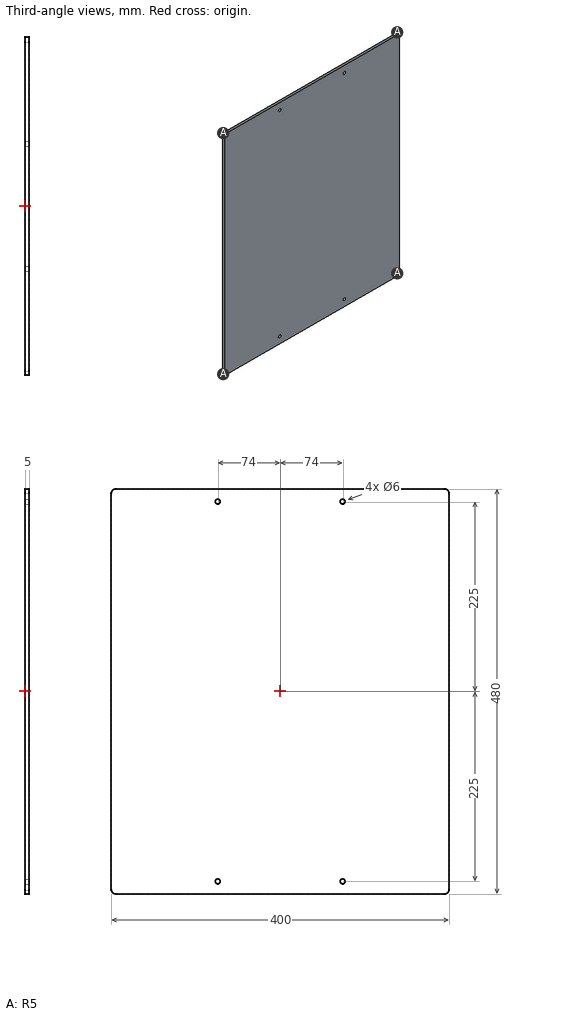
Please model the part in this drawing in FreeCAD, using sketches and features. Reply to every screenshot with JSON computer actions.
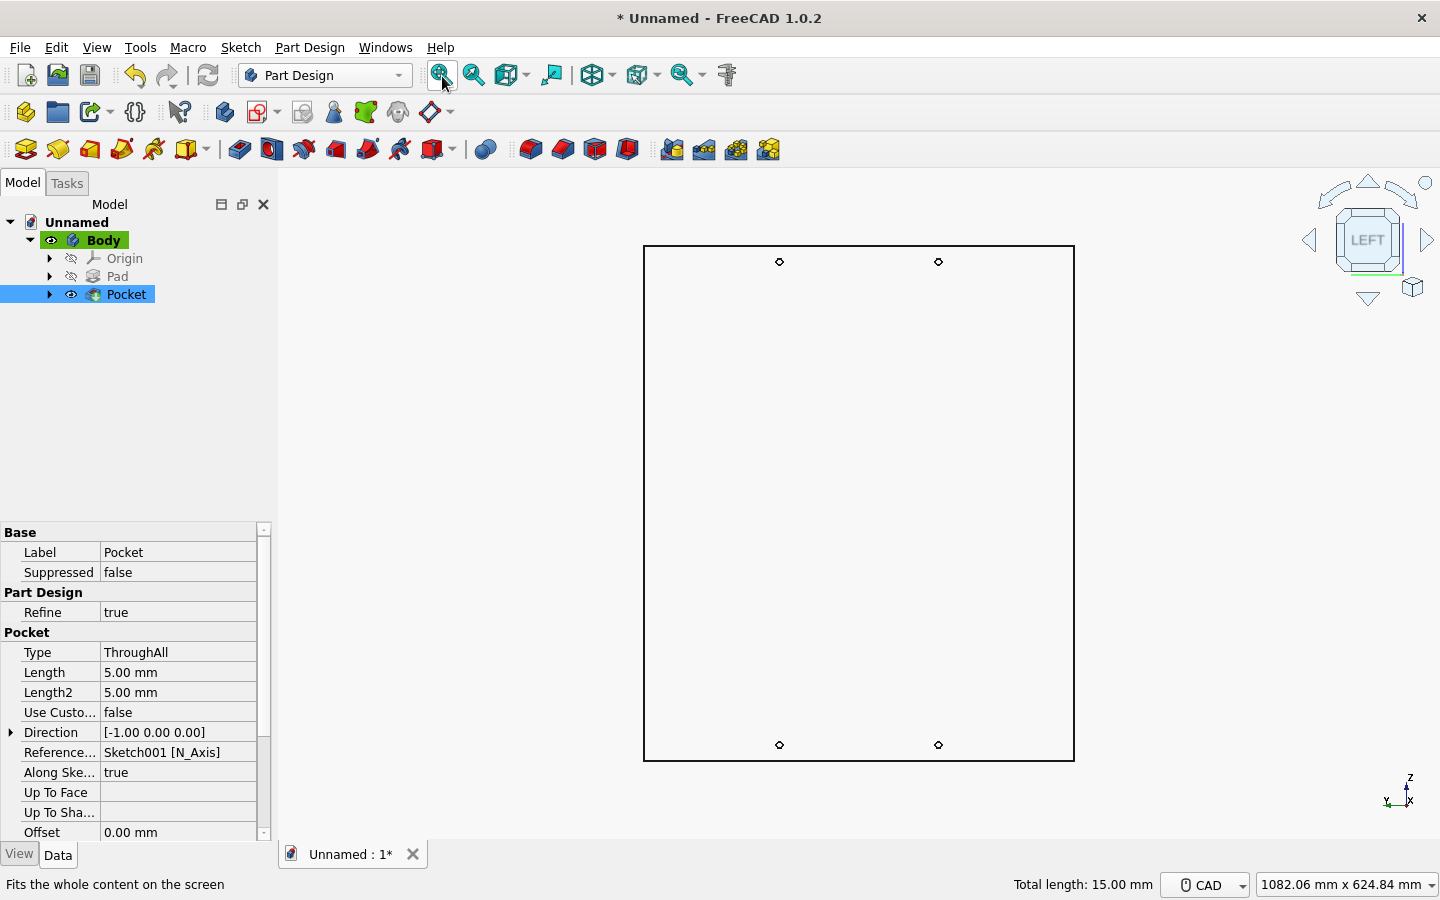
{"action": "key", "text": "0"}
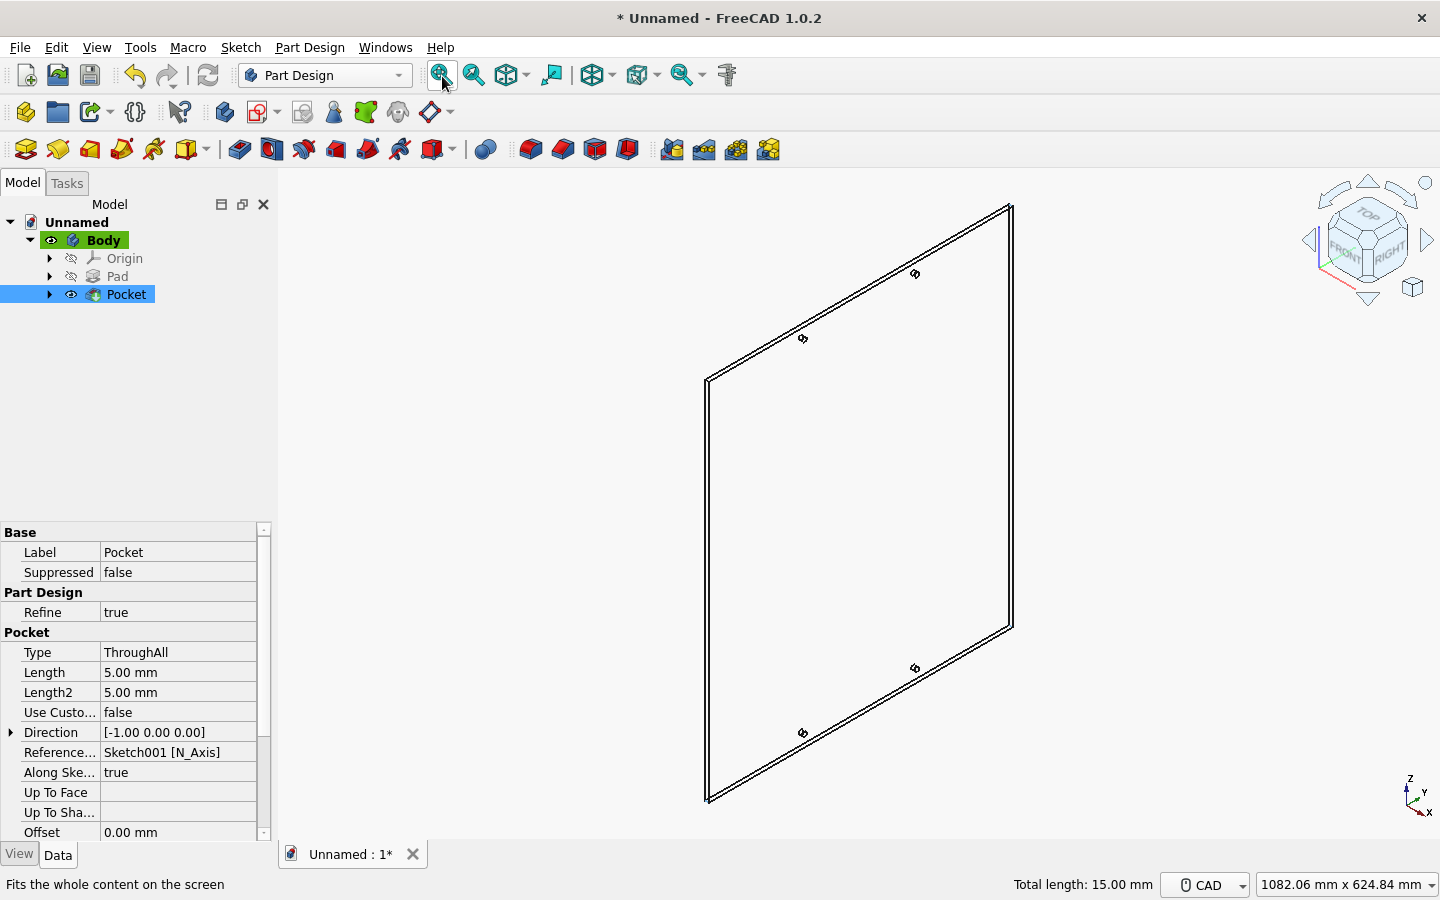
{"action": "scroll", "coordinate": [707, 380], "scroll_direction": "up", "scroll_amount": 11}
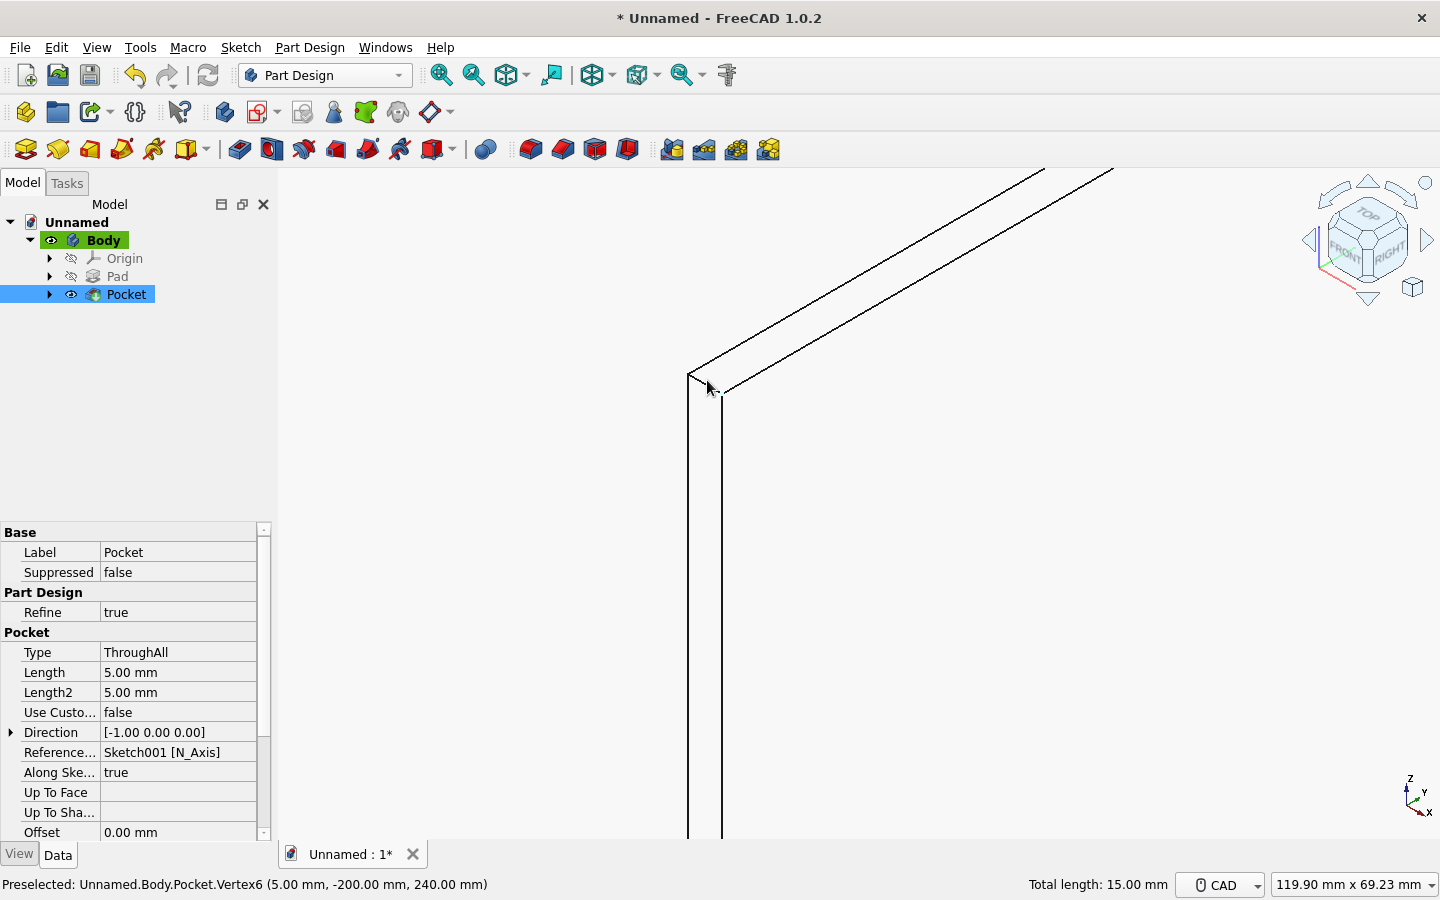
{"action": "left_click", "coordinate": [705, 383], "text": "ctrl"}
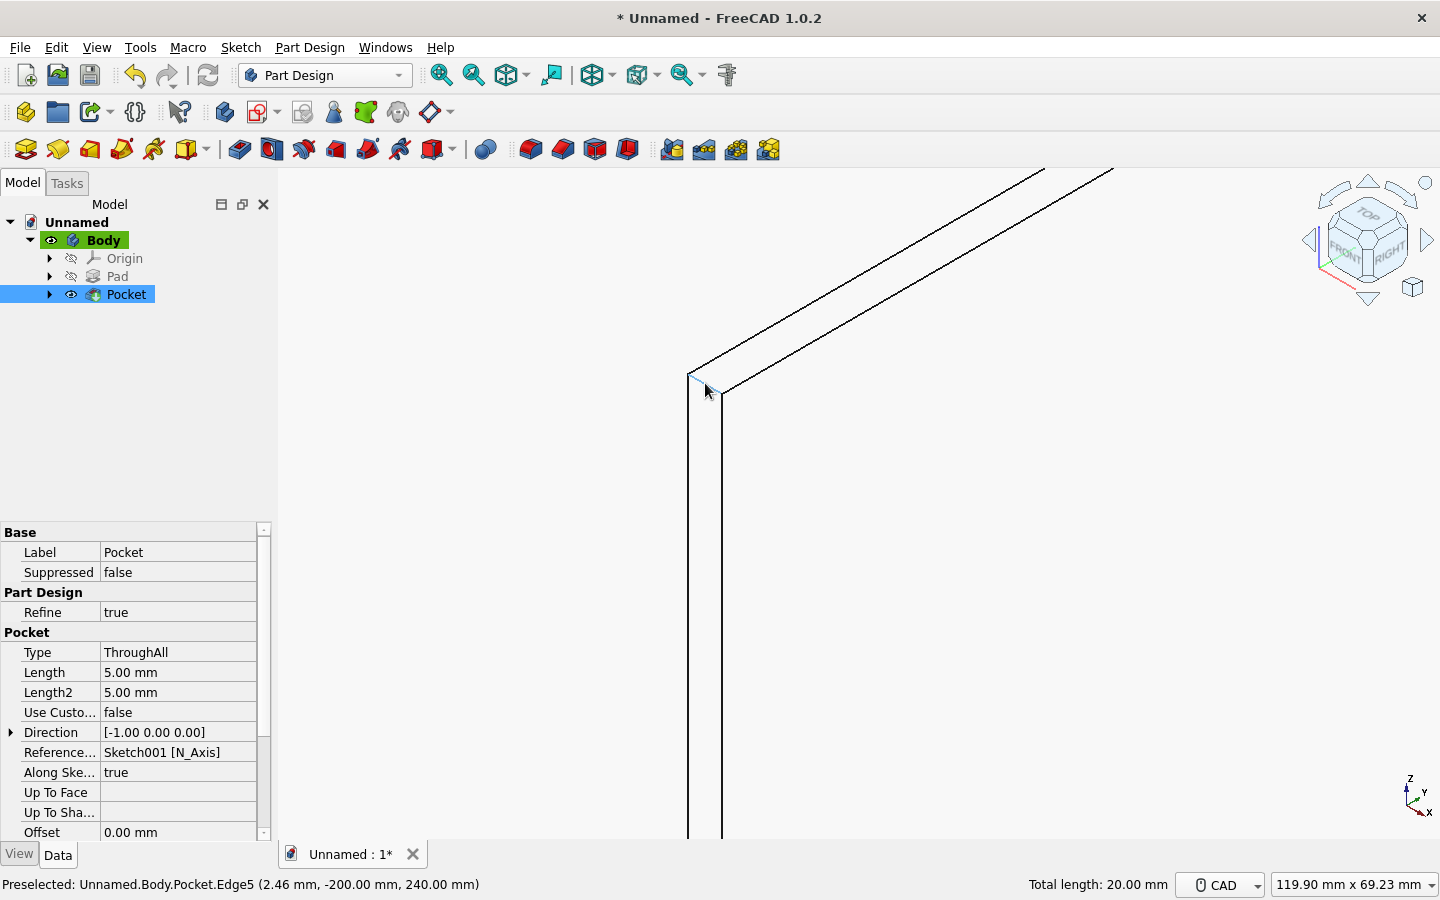
{"action": "key", "text": "v 1"}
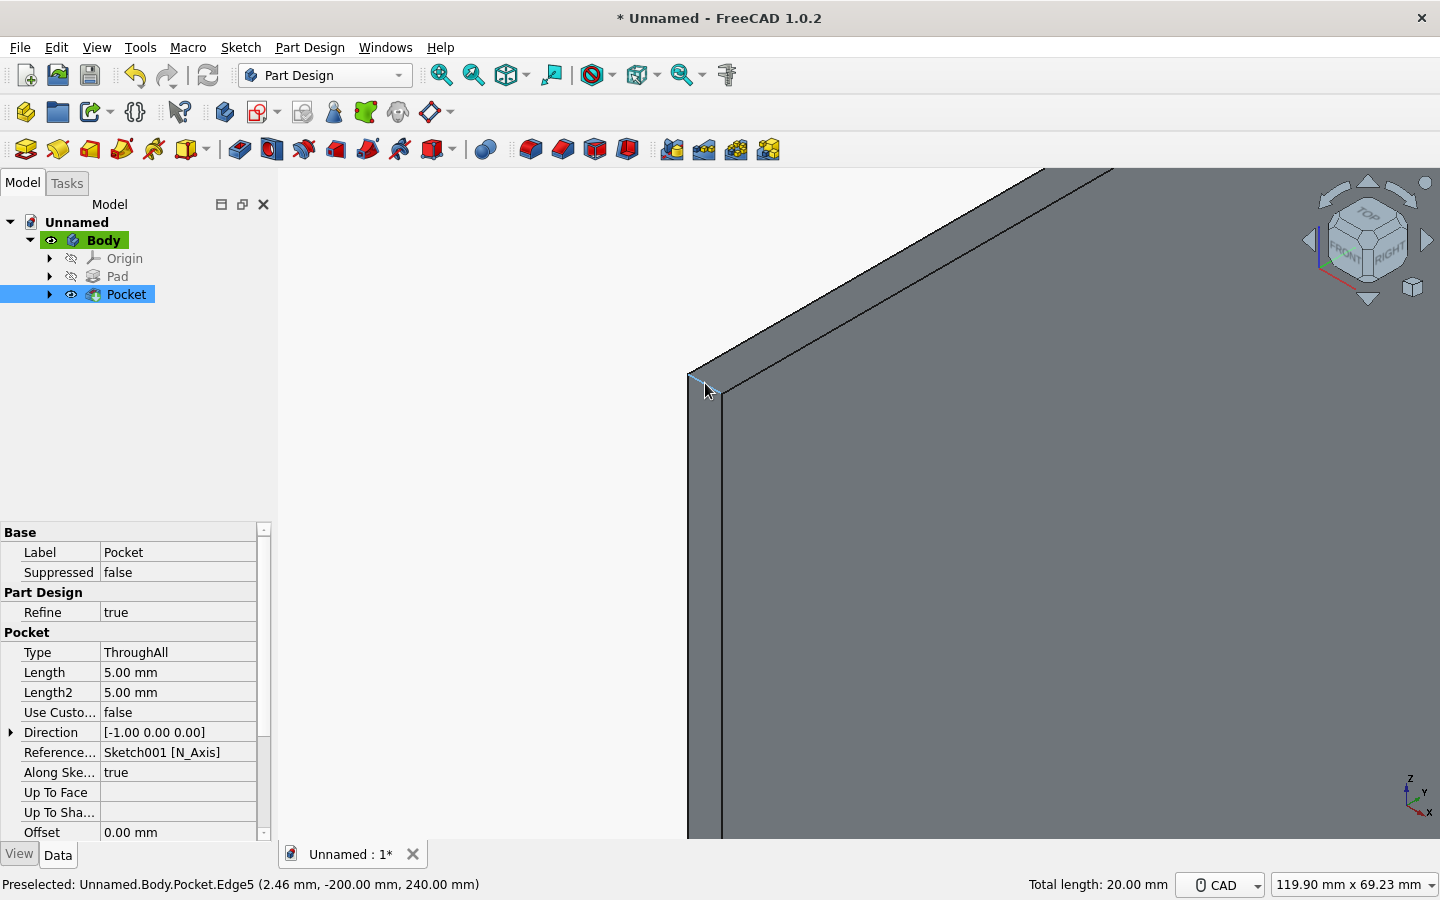
{"action": "left_click", "coordinate": [532, 150]}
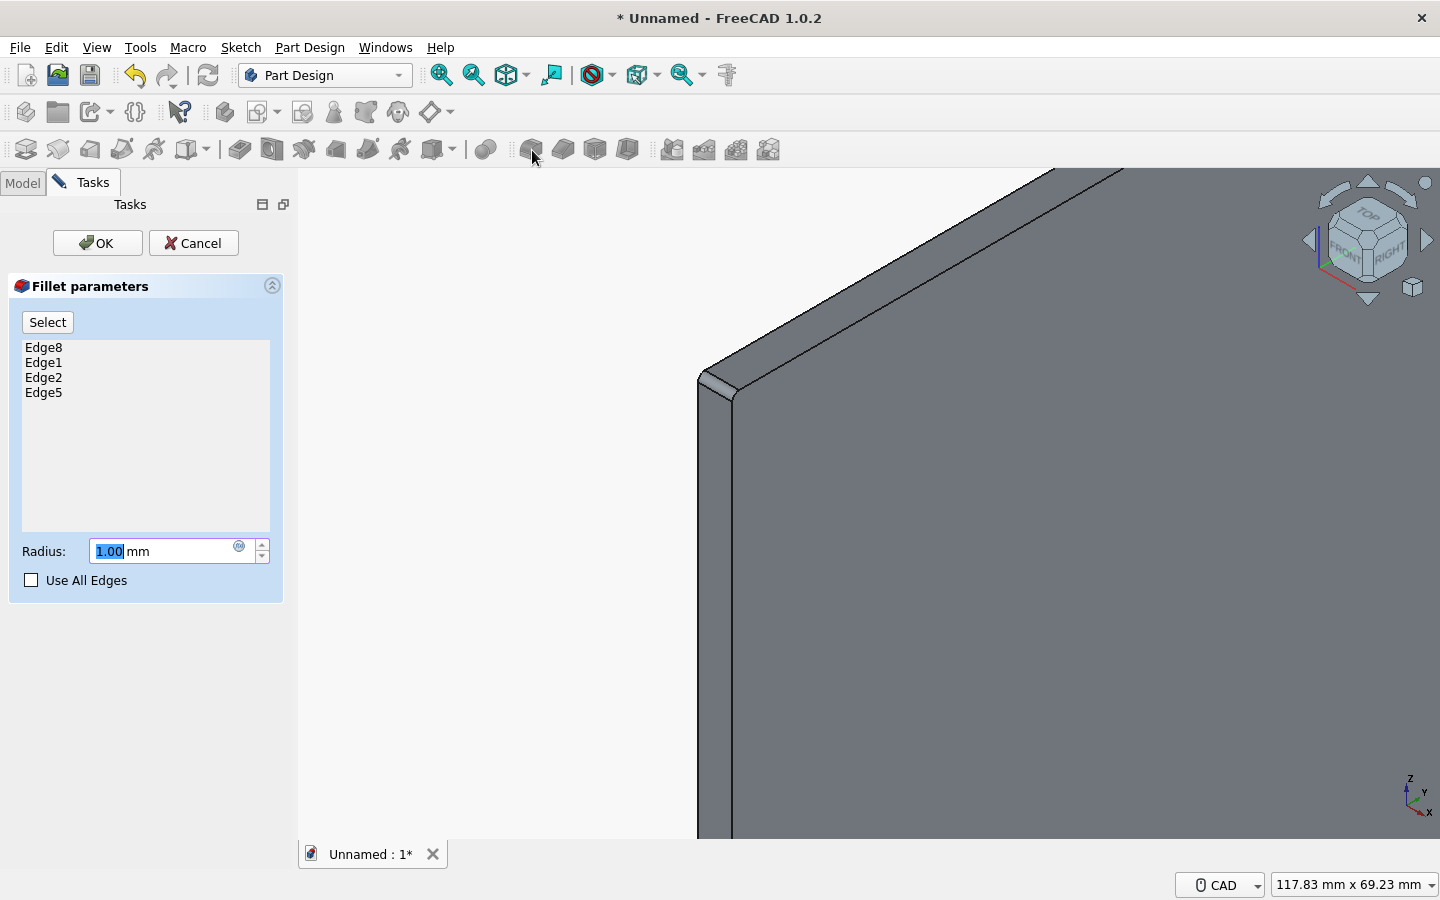
{"action": "type", "text": "5"}
{"action": "key", "text": "Tab"}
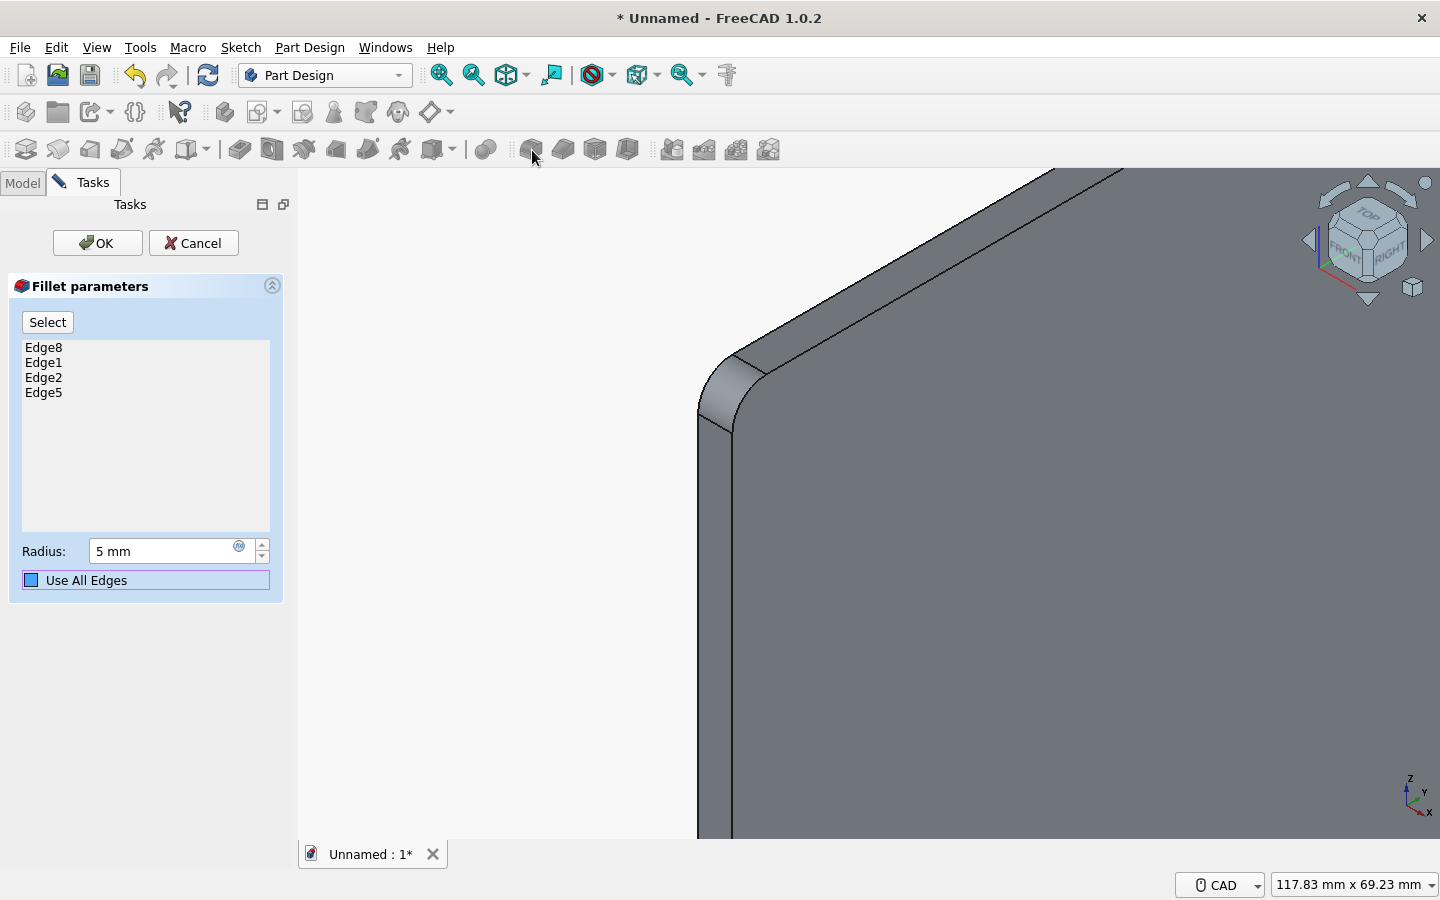
{"action": "left_click", "coordinate": [98, 243]}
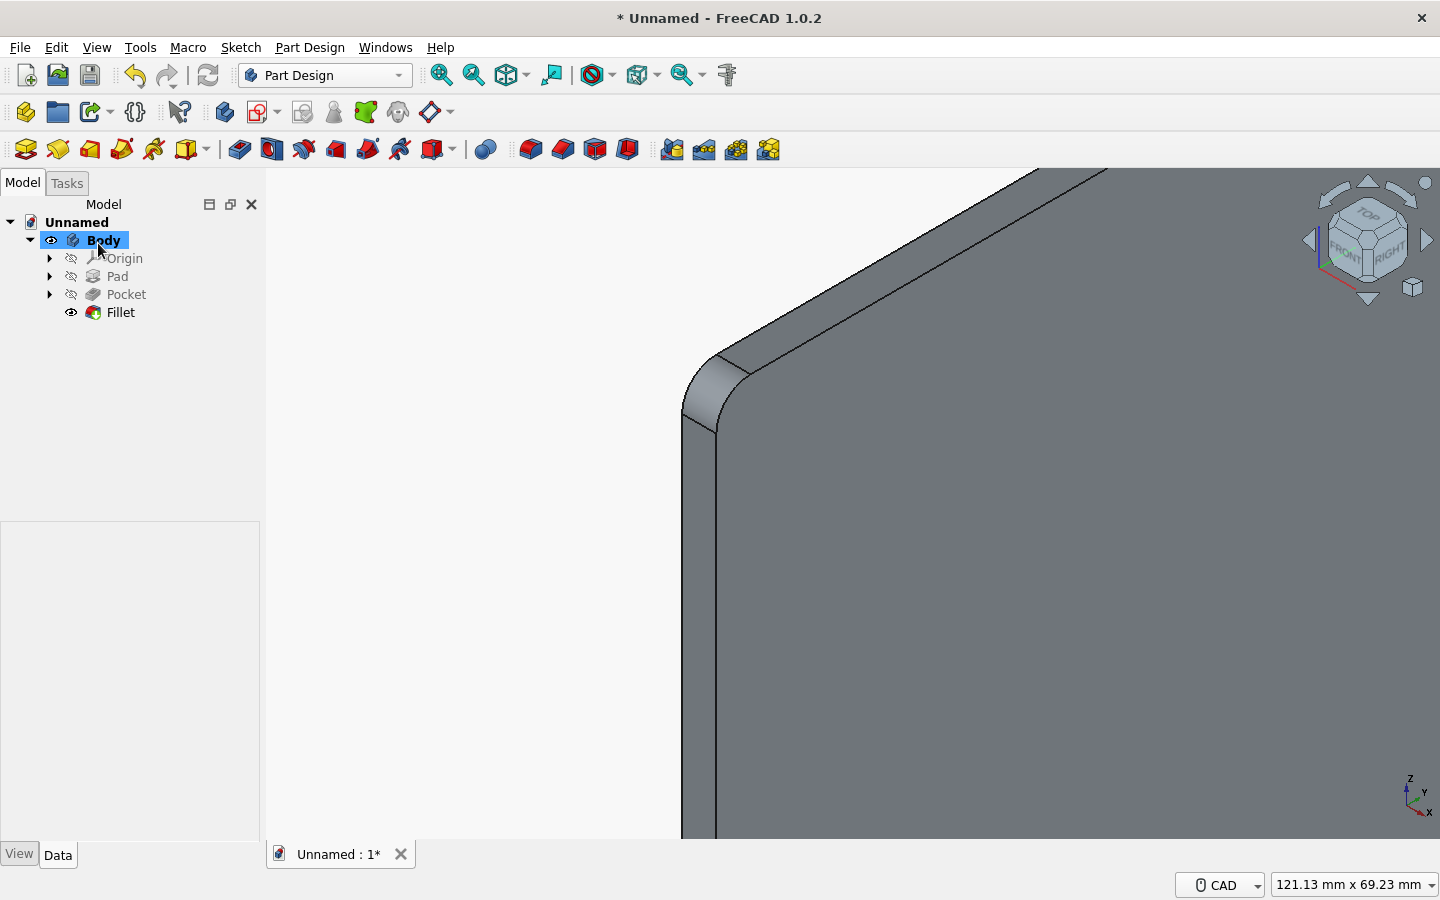
{"action": "left_click", "coordinate": [442, 76]}